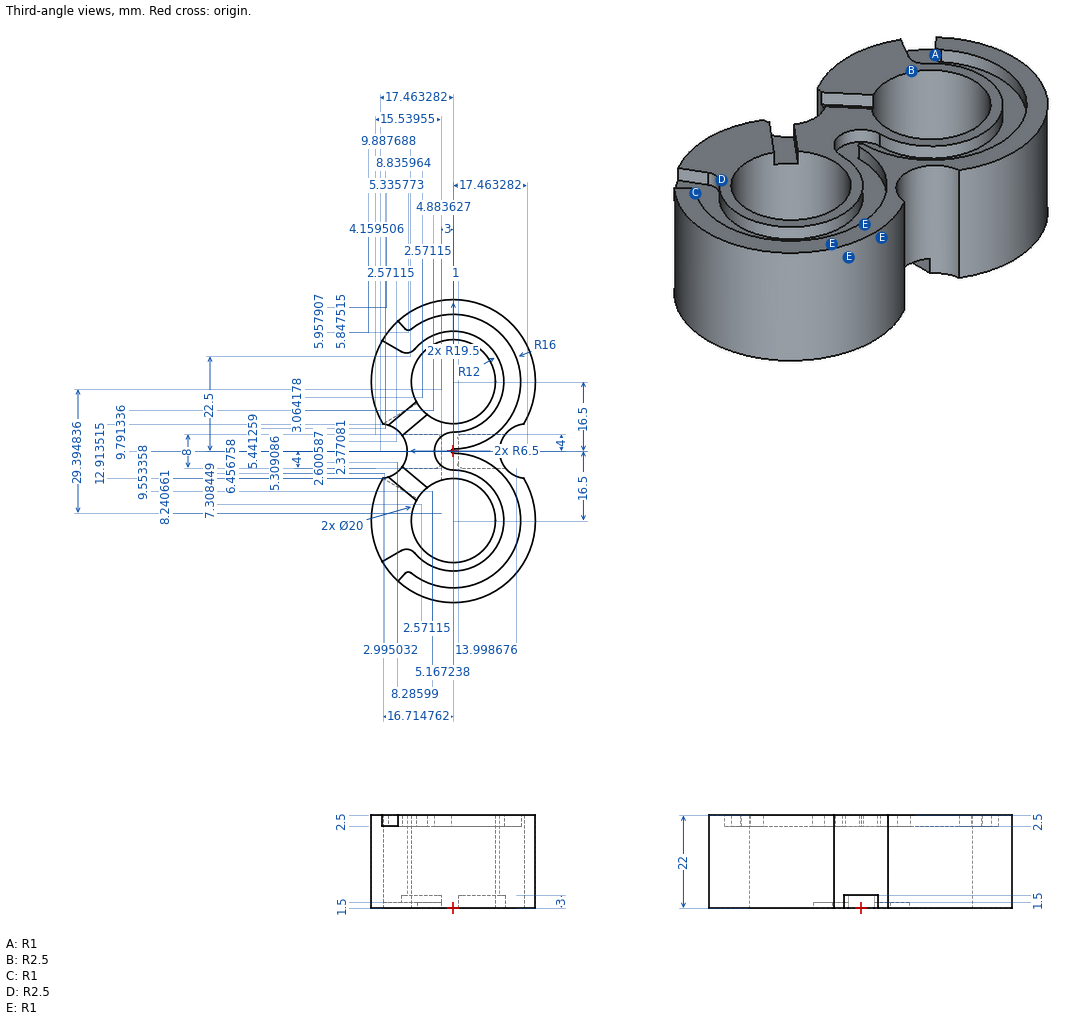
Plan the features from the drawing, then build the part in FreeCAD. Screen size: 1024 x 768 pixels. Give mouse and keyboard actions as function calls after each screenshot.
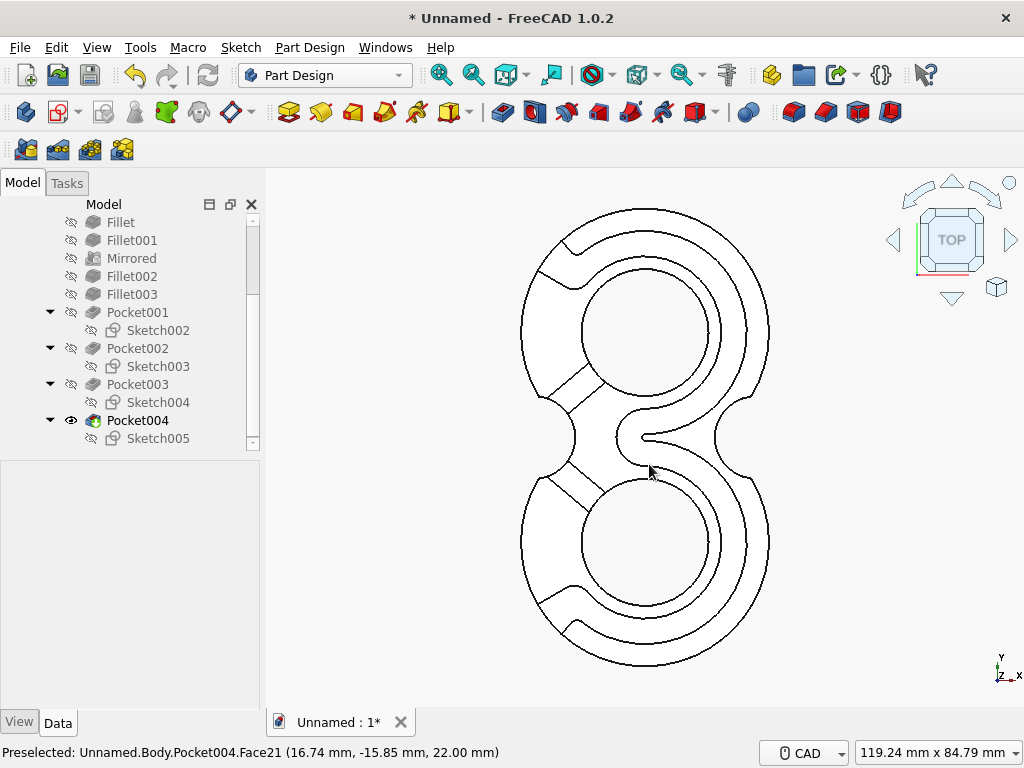
scroll(626, 411, up, 8)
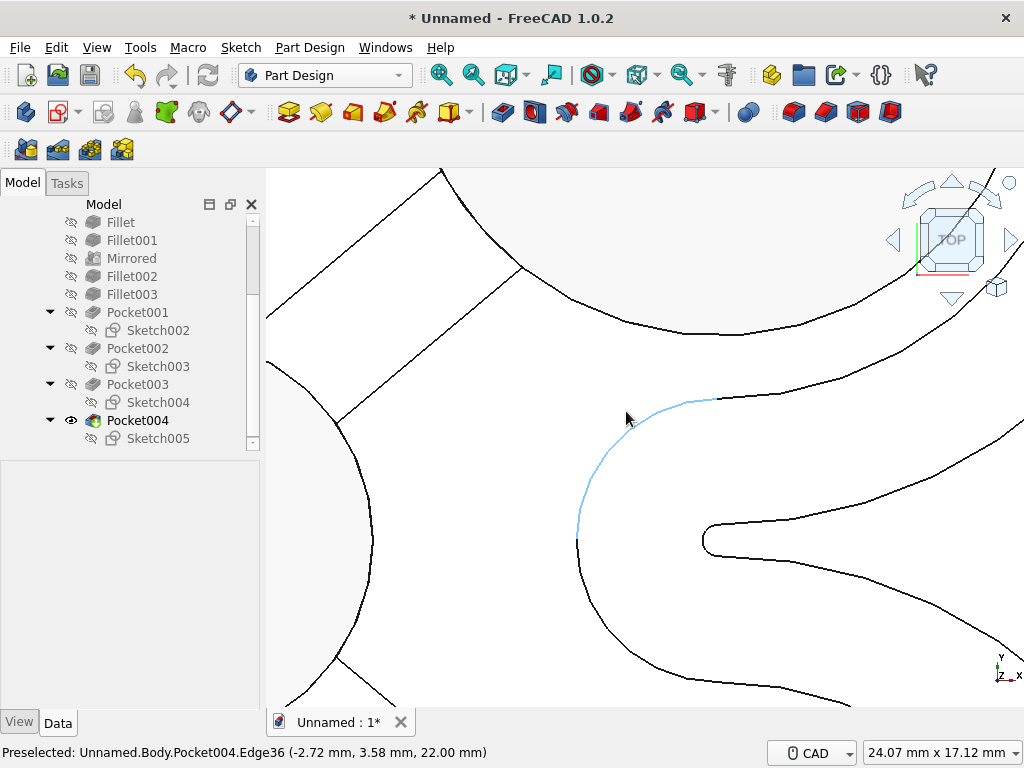
click(442, 76)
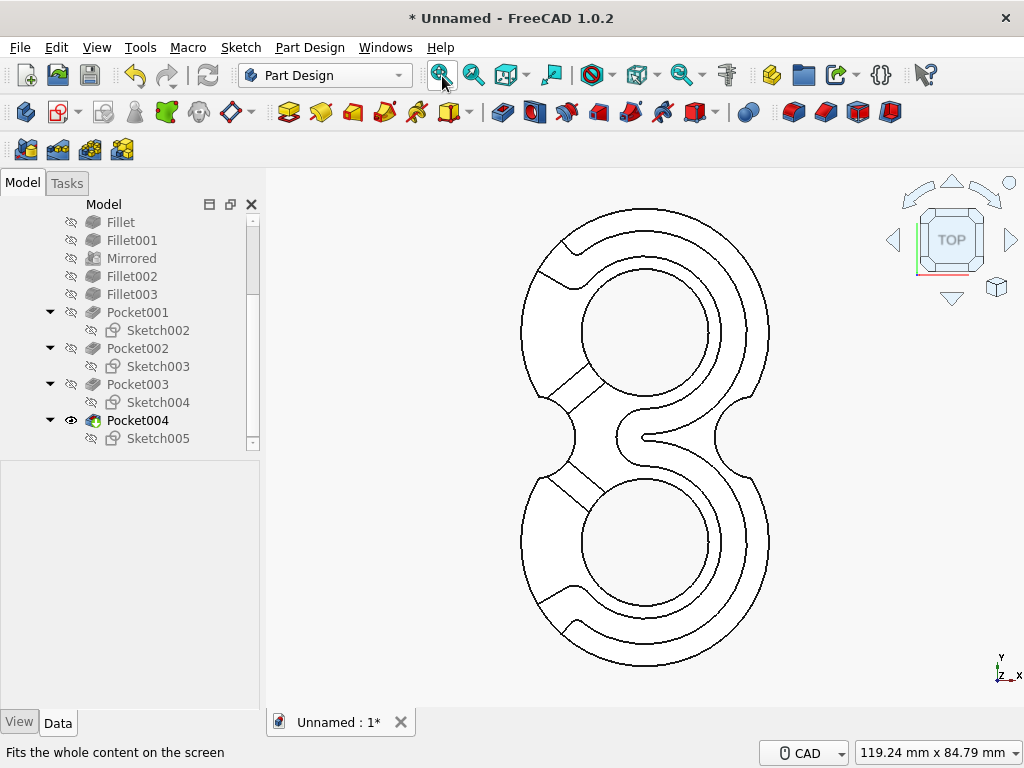
key(1)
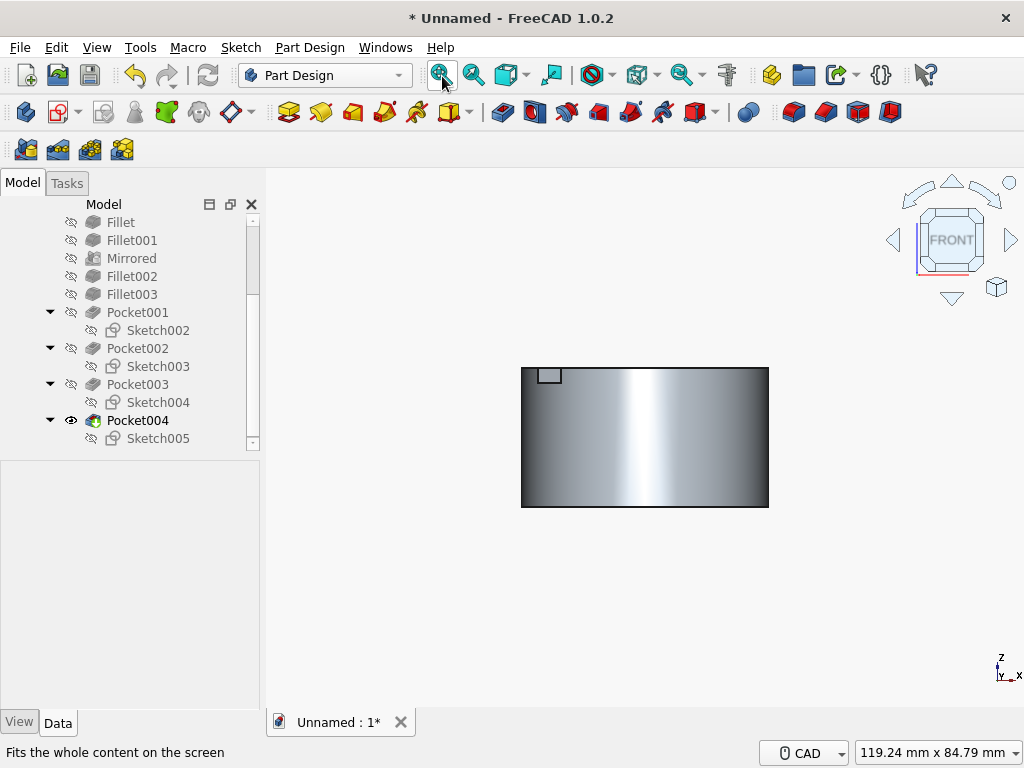
click(442, 76)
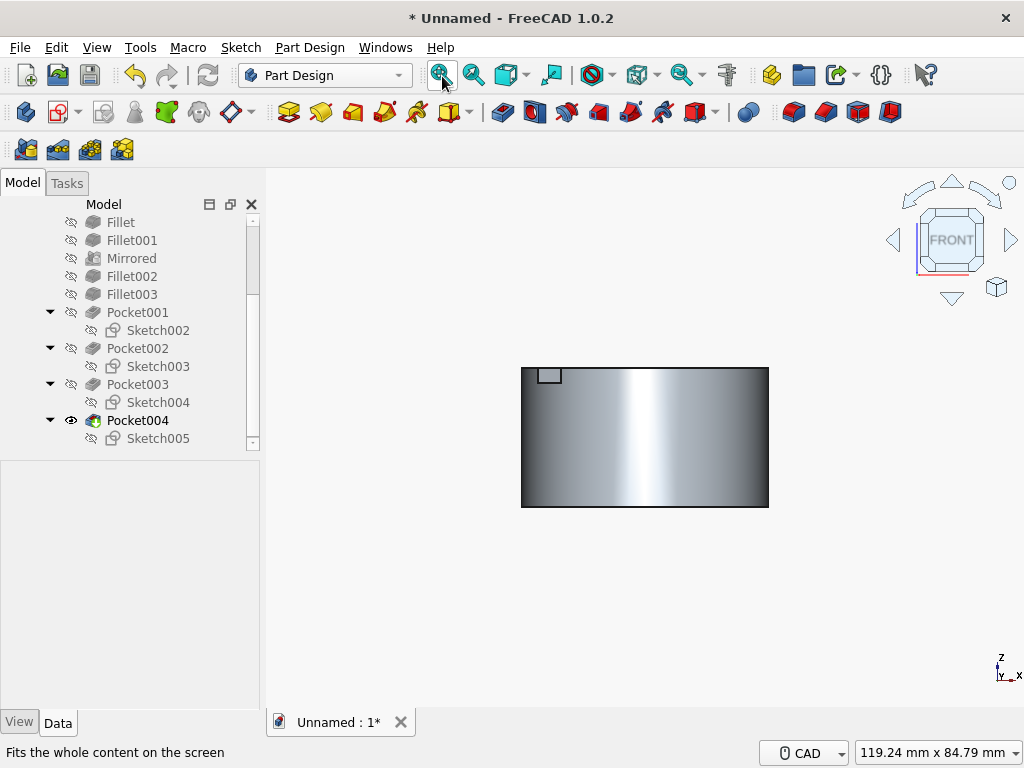
scroll(626, 492, up, 8)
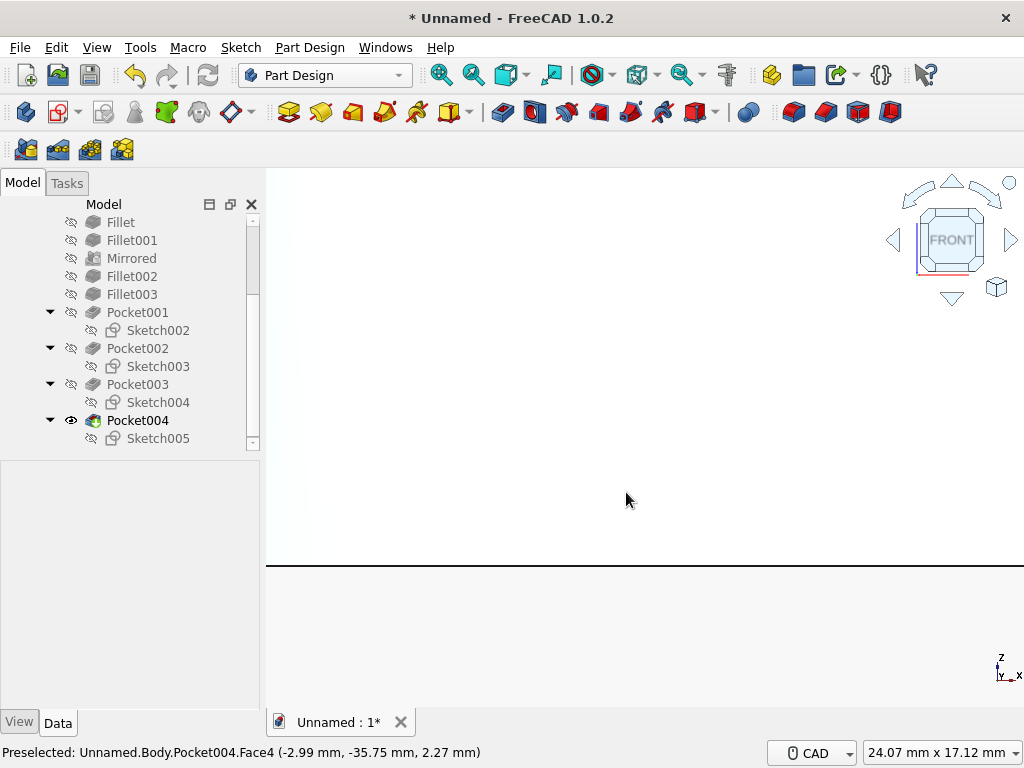
click(442, 76)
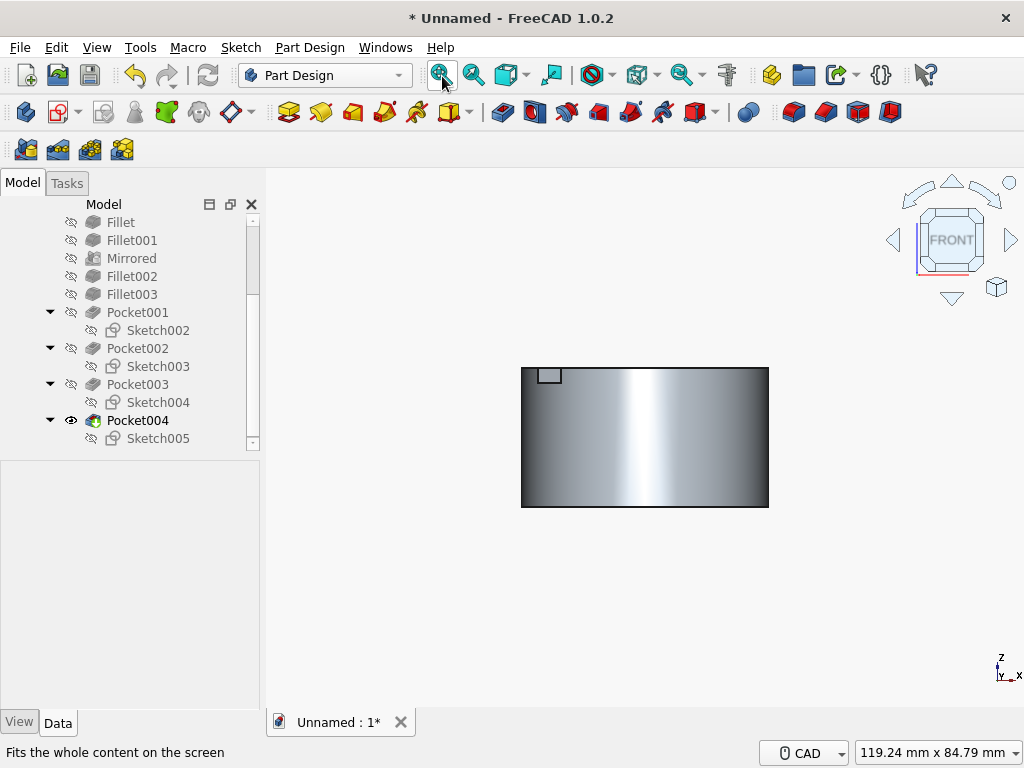
key(3)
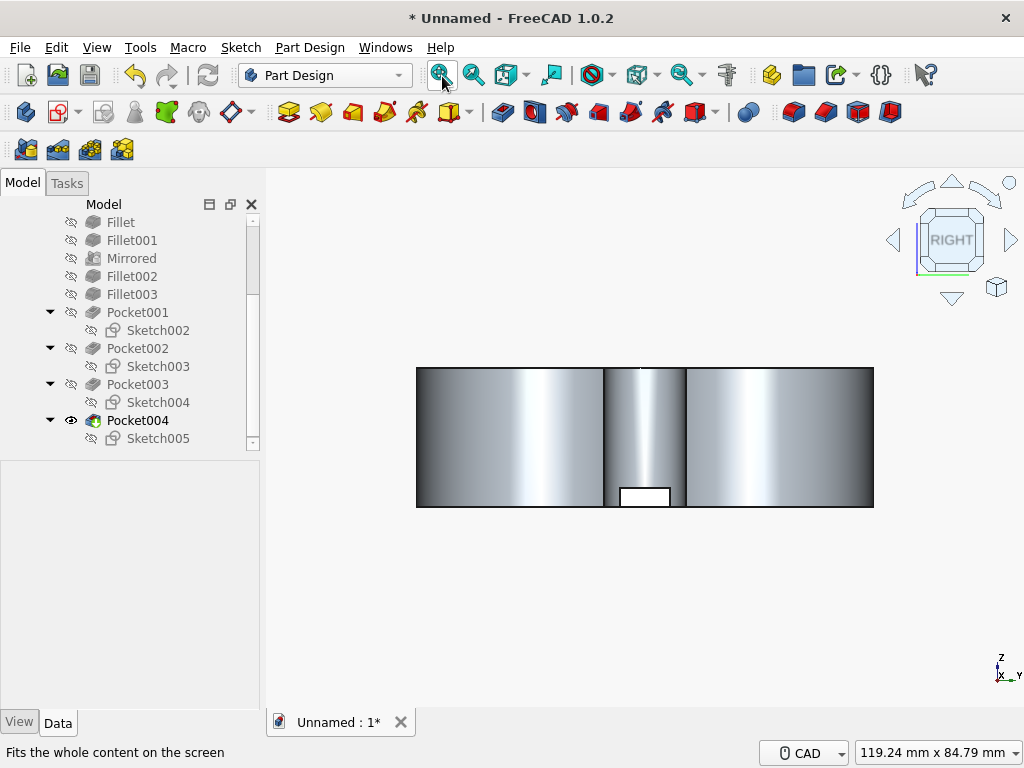
scroll(670, 492, up, 8)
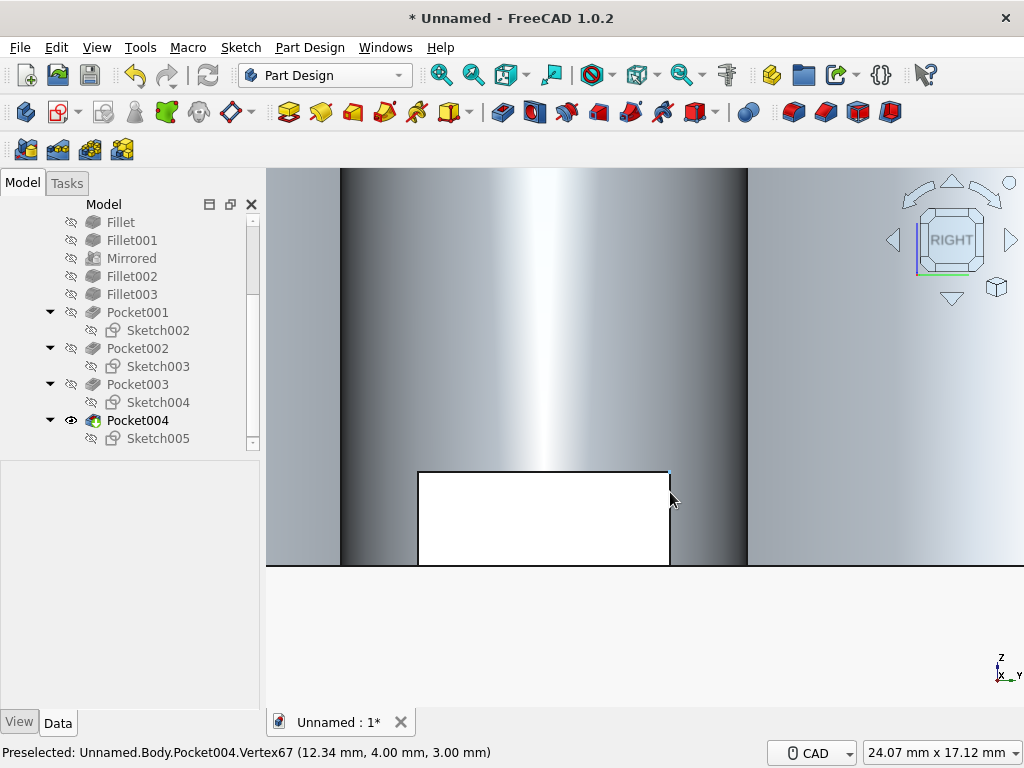
click(442, 76)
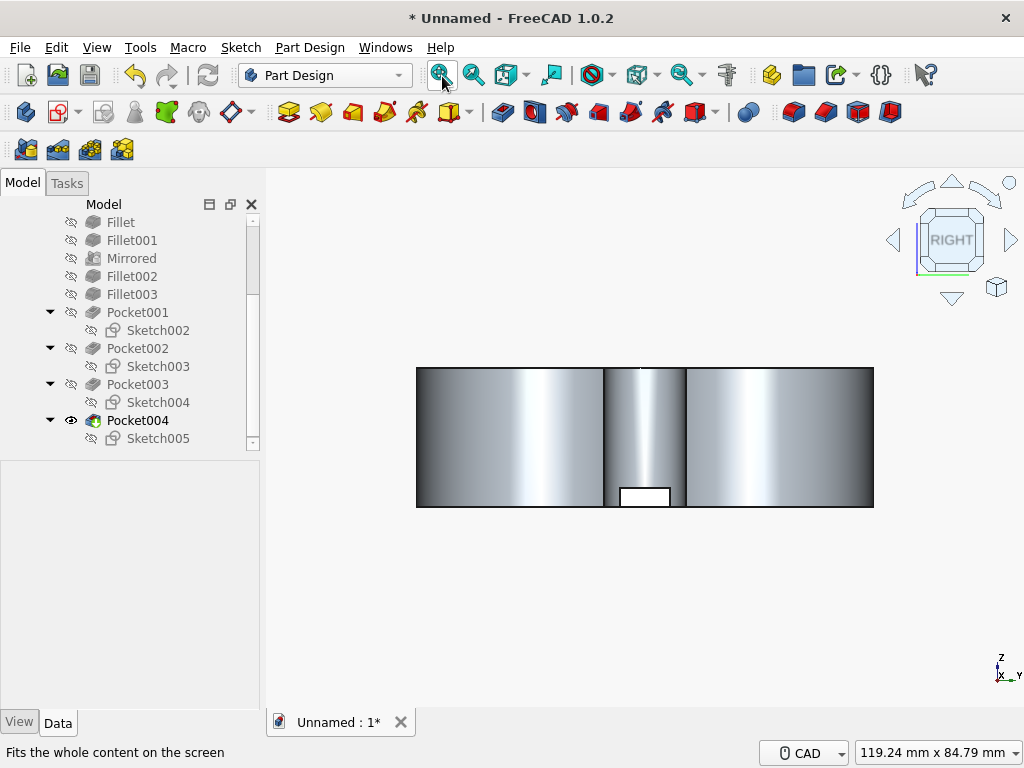
key(5)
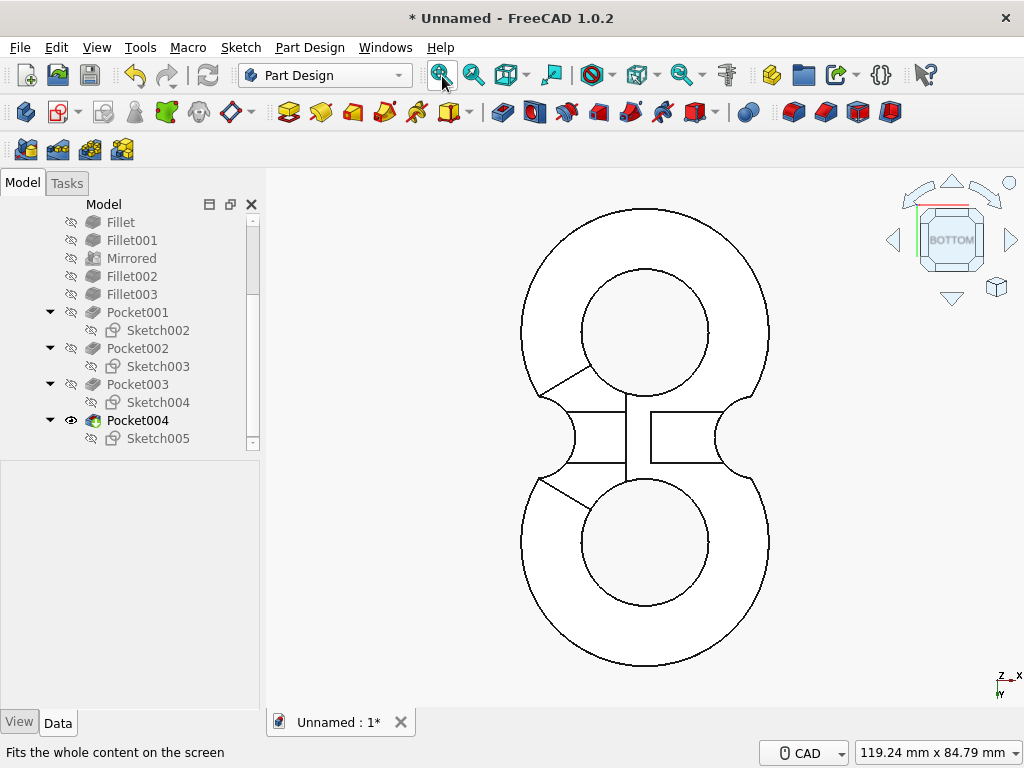
scroll(626, 462, up, 8)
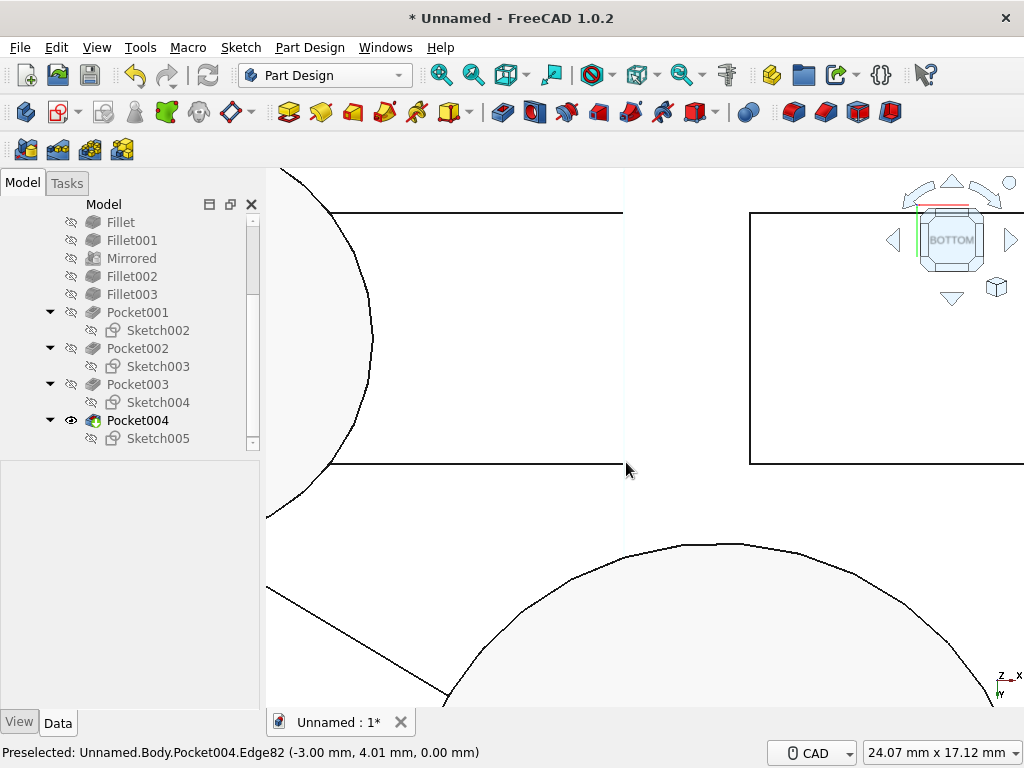
click(442, 76)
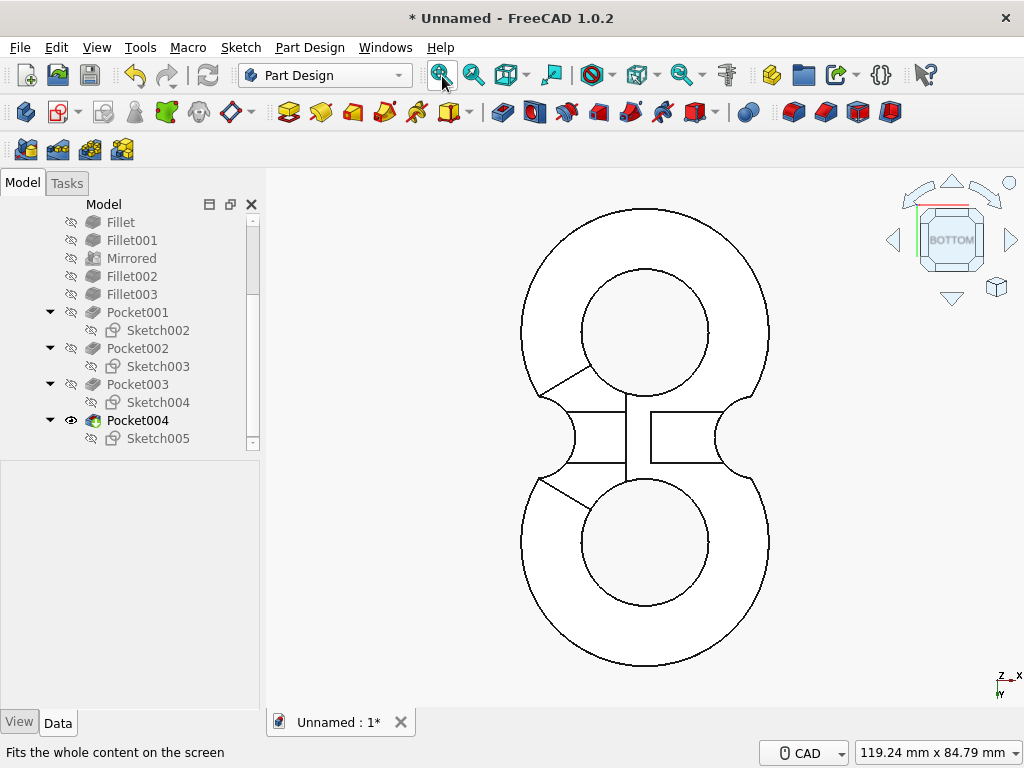
key(4)